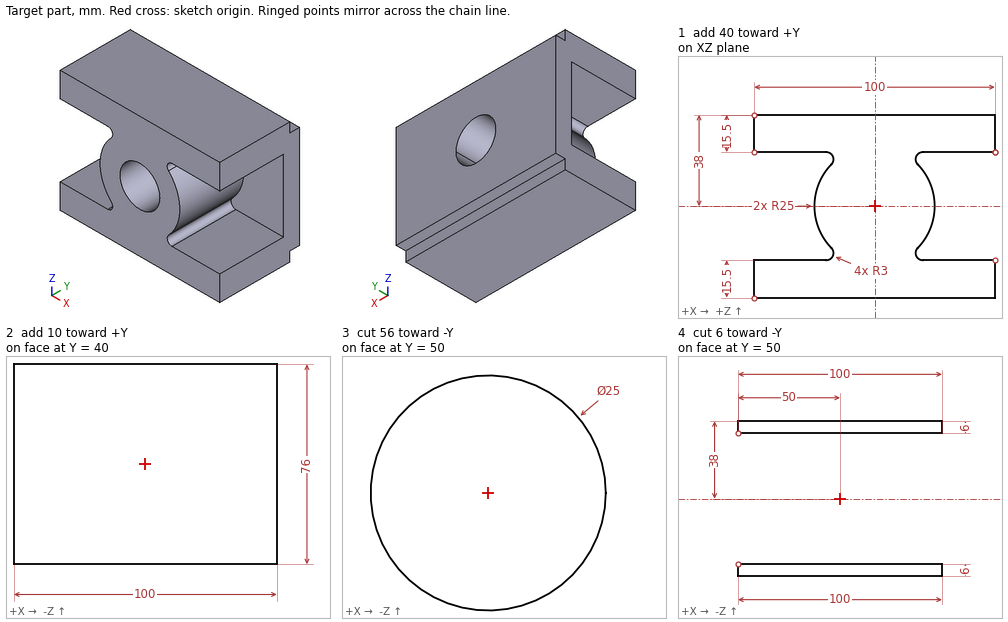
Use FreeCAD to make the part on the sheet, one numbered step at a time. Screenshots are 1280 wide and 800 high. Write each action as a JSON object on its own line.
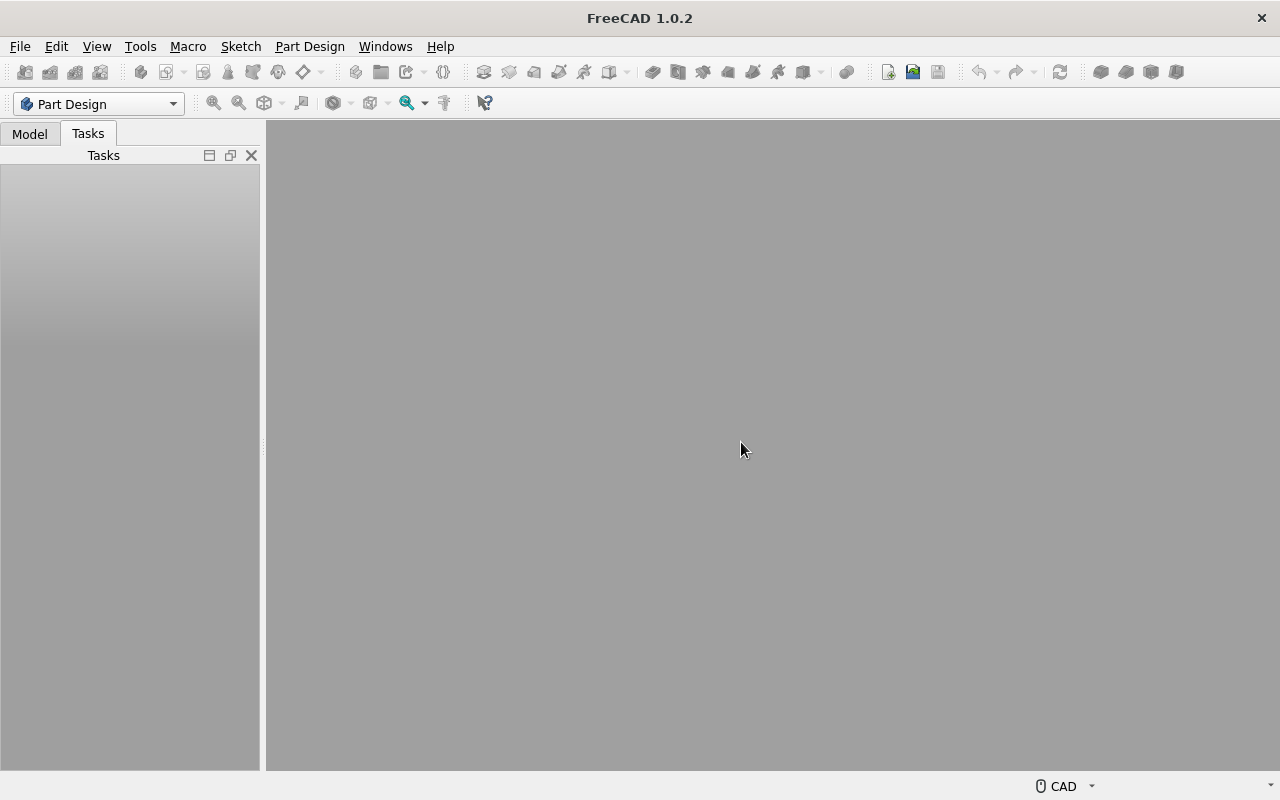
{"action": "left_click", "coordinate": [888, 72]}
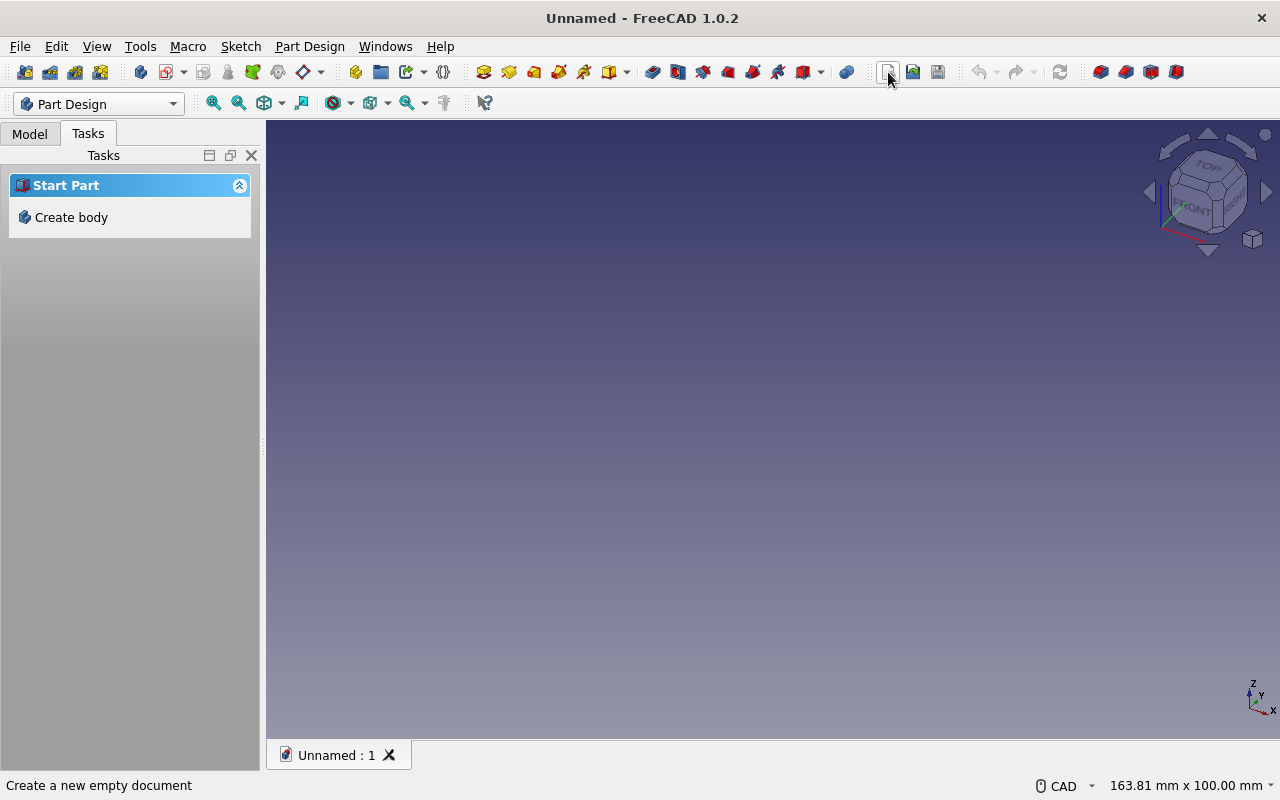
{"action": "left_click", "coordinate": [166, 72]}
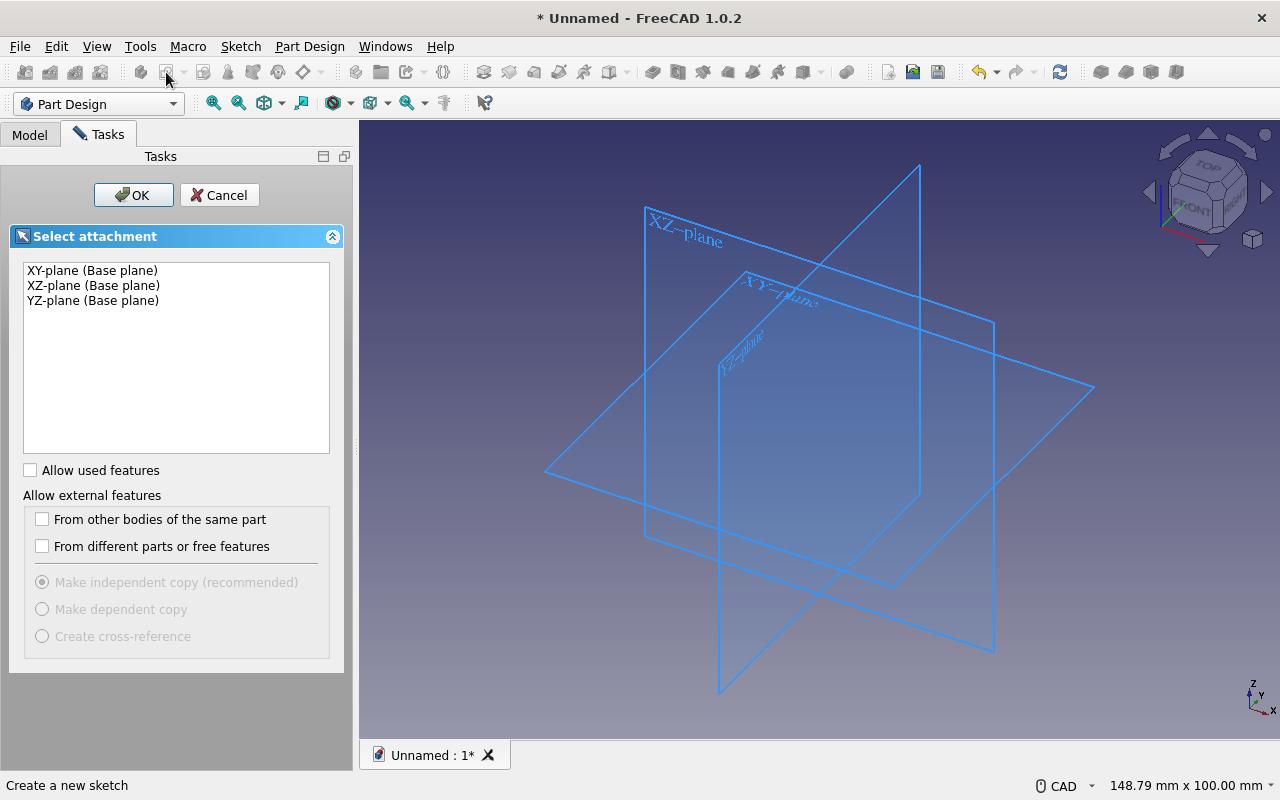
{"action": "left_click", "coordinate": [84, 286]}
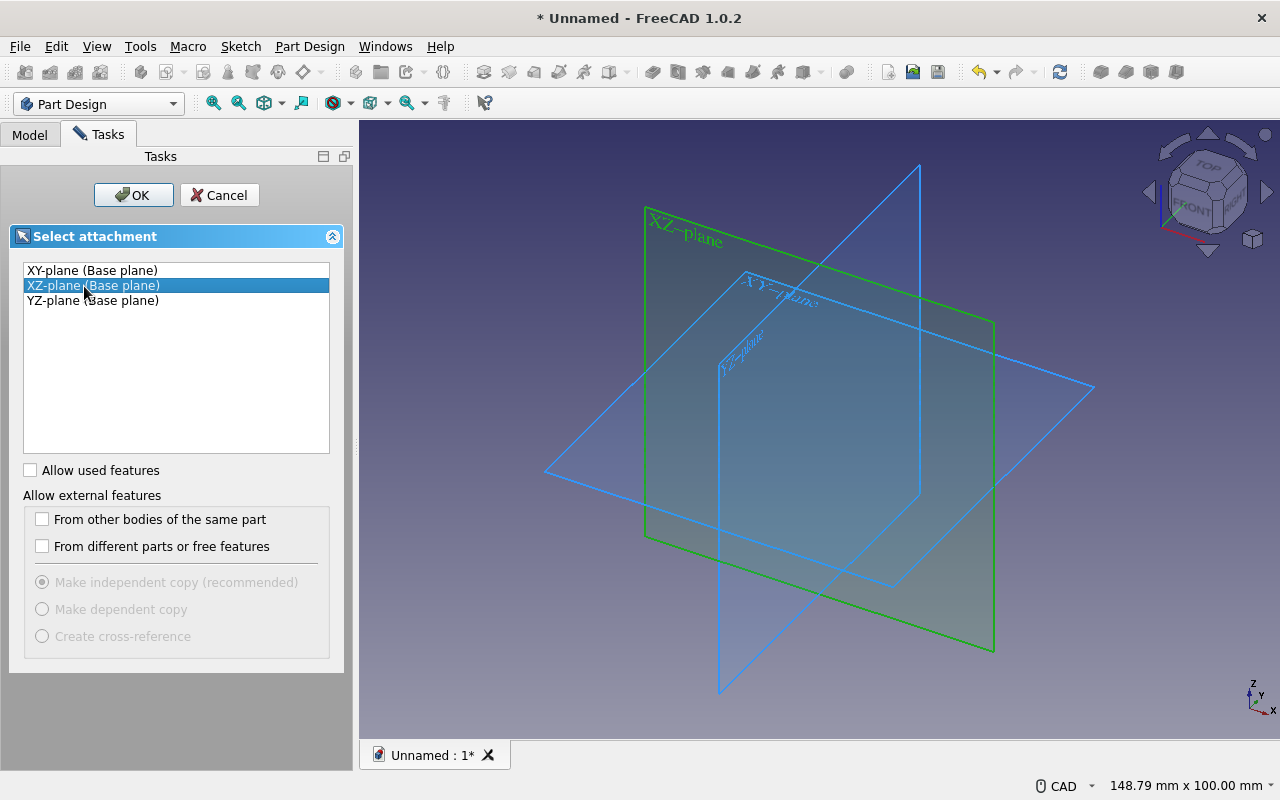
{"action": "left_click", "coordinate": [134, 195]}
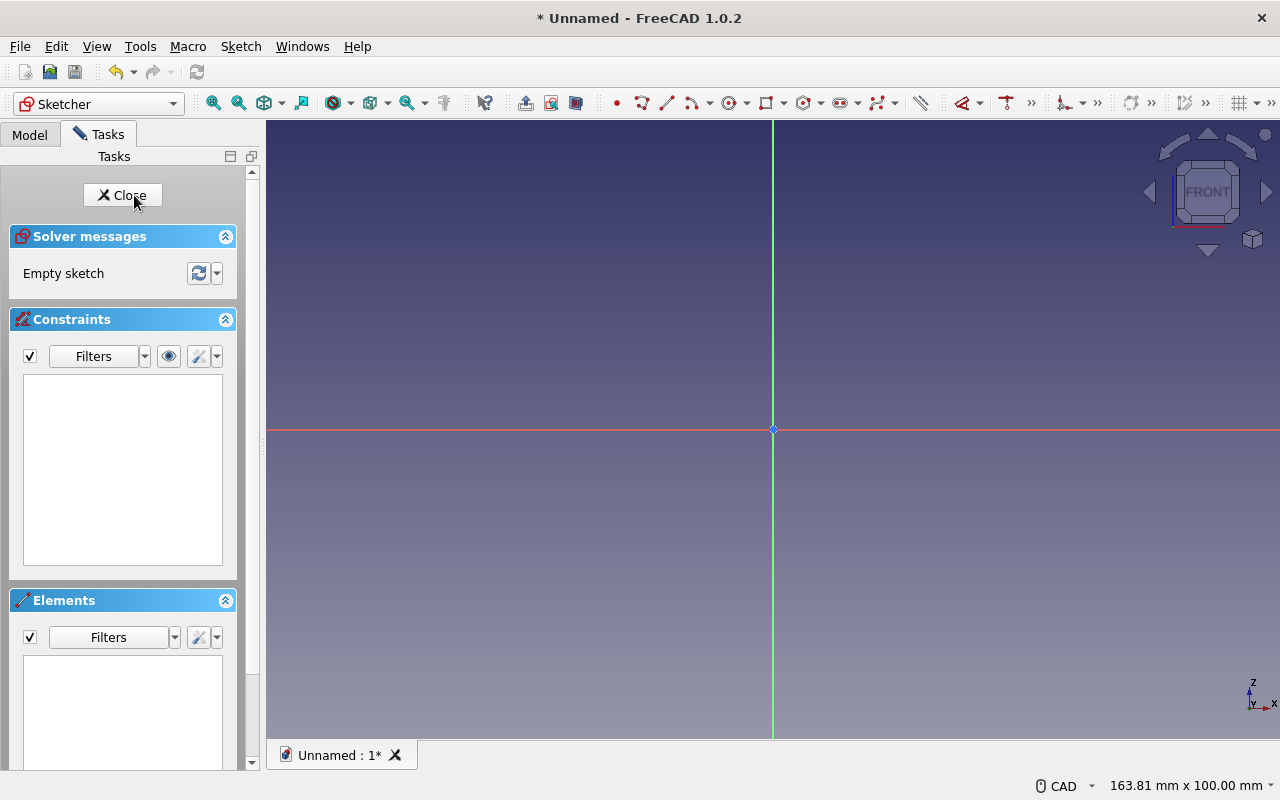
{"action": "left_click", "coordinate": [642, 104]}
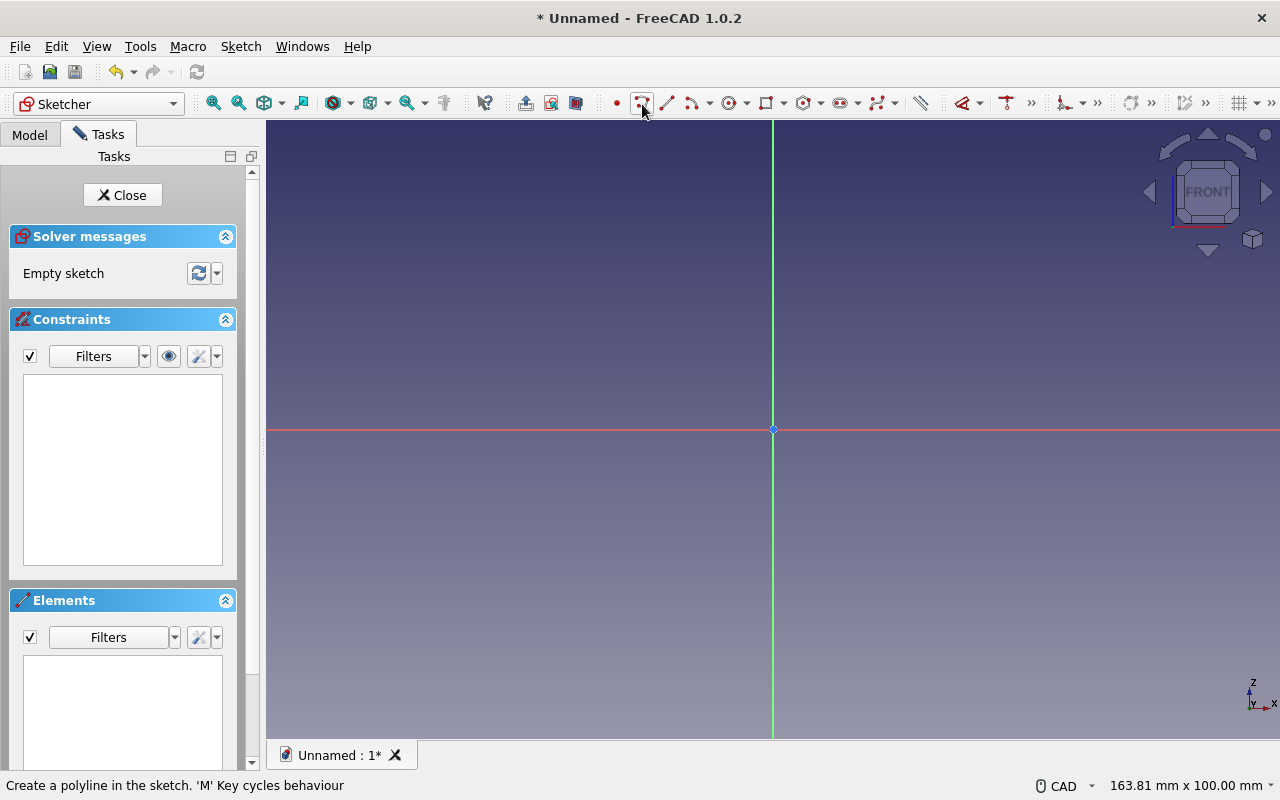
{"action": "left_click", "coordinate": [649, 290]}
{"action": "left_click", "coordinate": [464, 290]}
{"action": "left_click", "coordinate": [464, 194]}
{"action": "left_click", "coordinate": [1082, 194]}
{"action": "left_click", "coordinate": [1082, 290]}
{"action": "left_click", "coordinate": [897, 290]}
{"action": "right_click", "coordinate": [897, 290]}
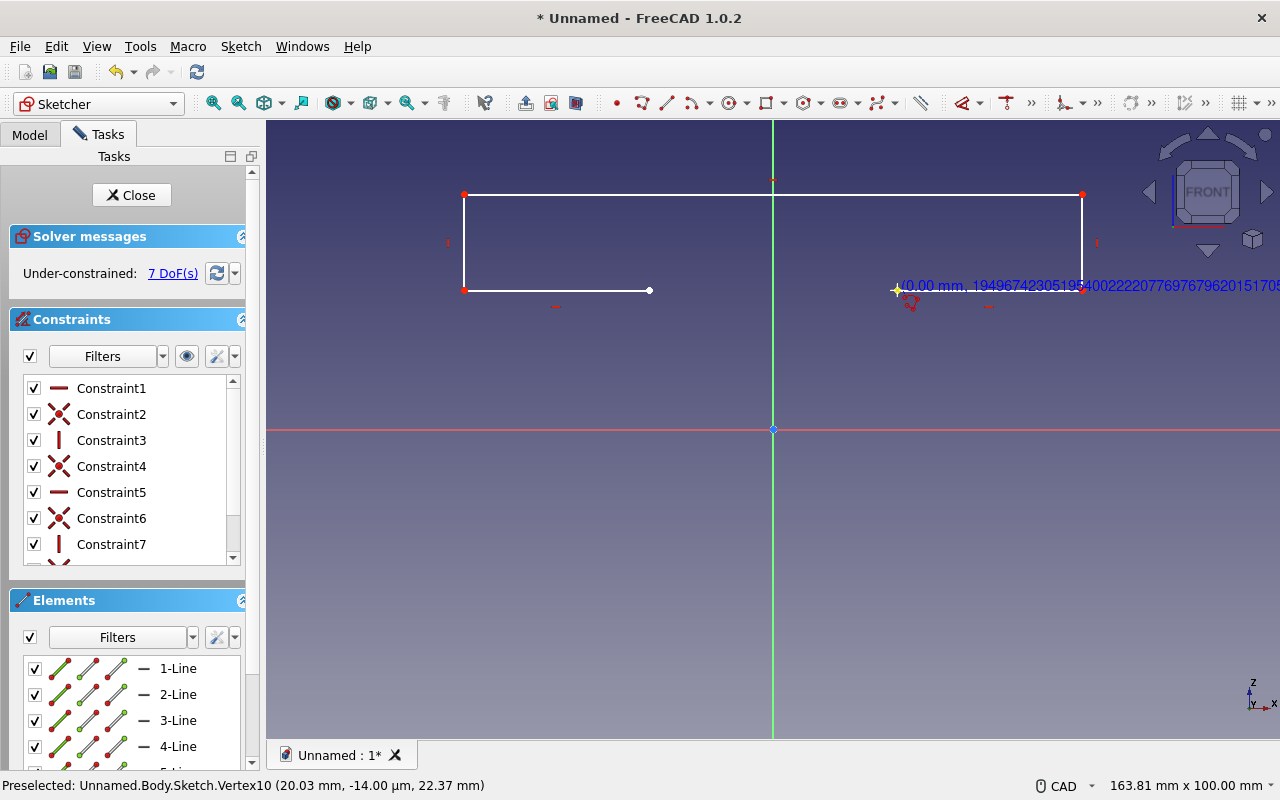
{"action": "left_click", "coordinate": [897, 569]}
{"action": "left_click", "coordinate": [1082, 569]}
{"action": "left_click", "coordinate": [1082, 665]}
{"action": "left_click", "coordinate": [464, 665]}
{"action": "left_click", "coordinate": [464, 569]}
{"action": "left_click", "coordinate": [649, 569]}
{"action": "right_click", "coordinate": [649, 569]}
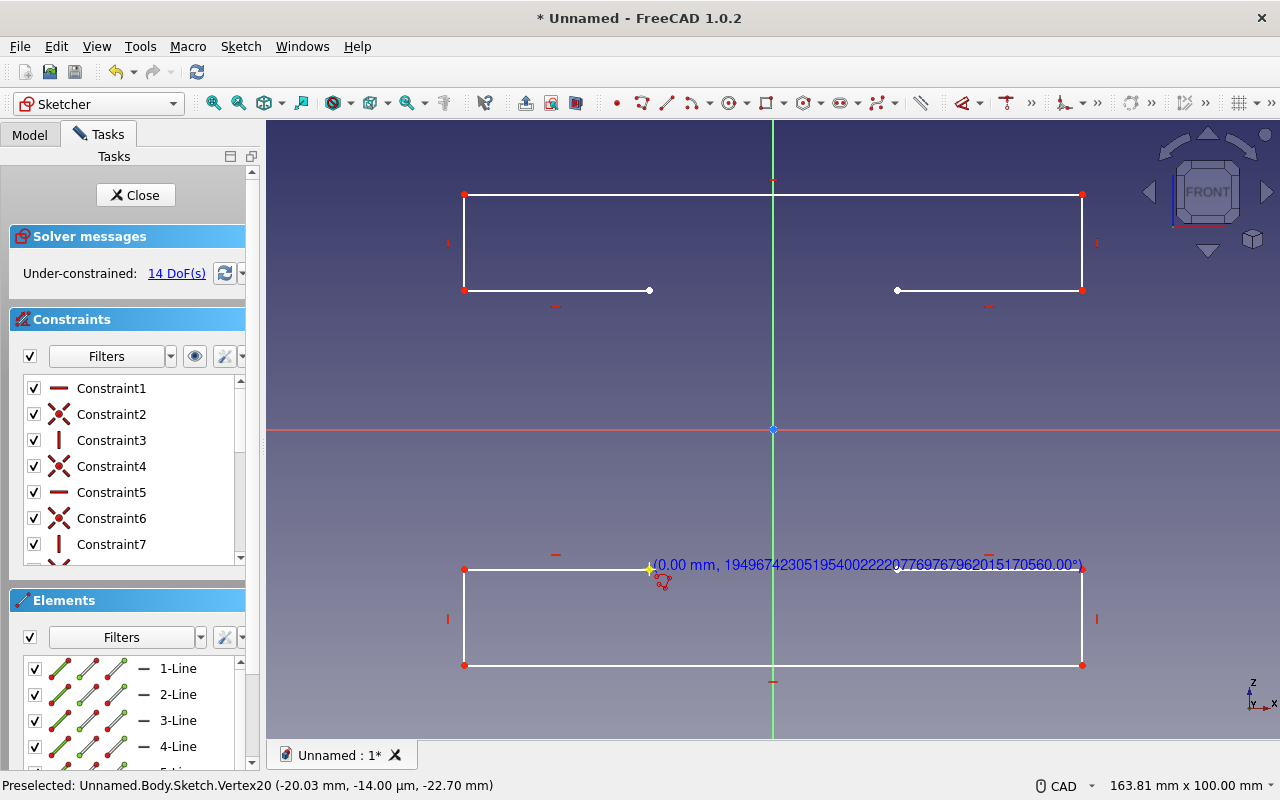
{"action": "left_click", "coordinate": [710, 104]}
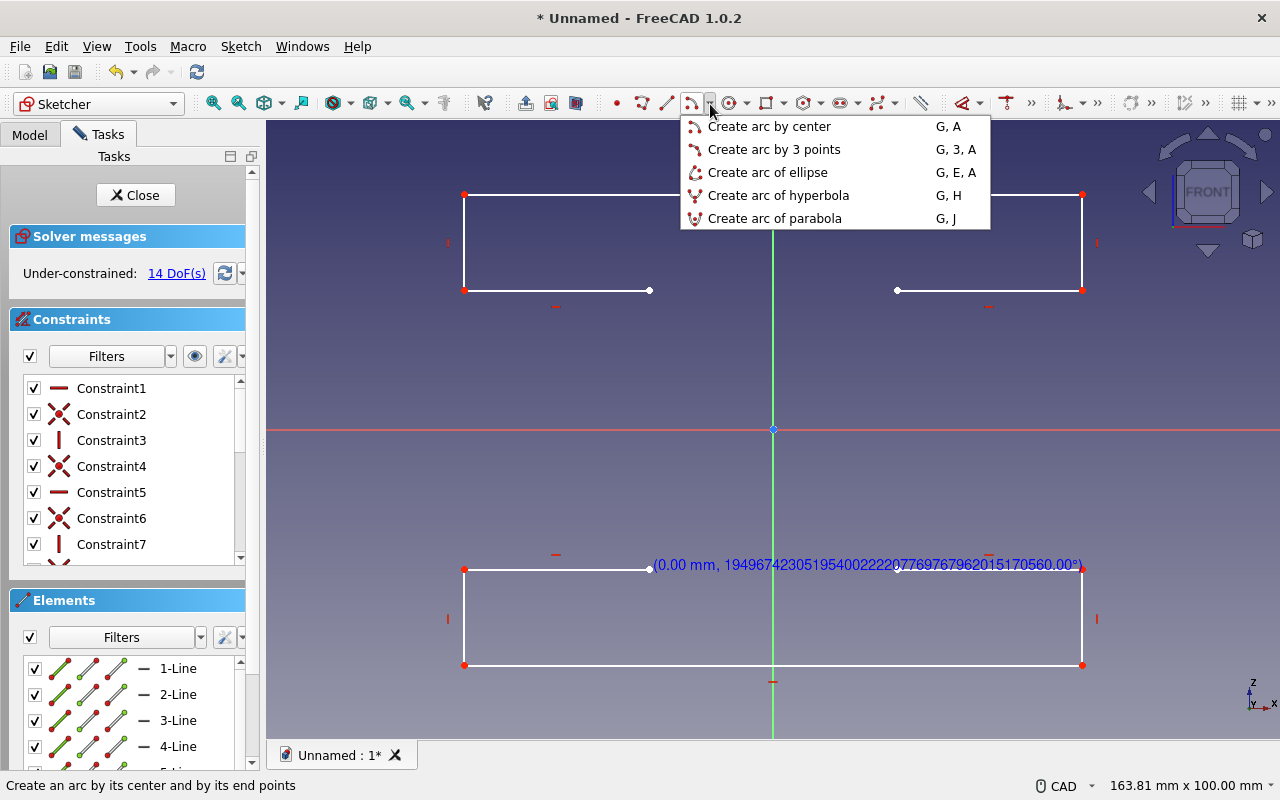
{"action": "left_click", "coordinate": [836, 150]}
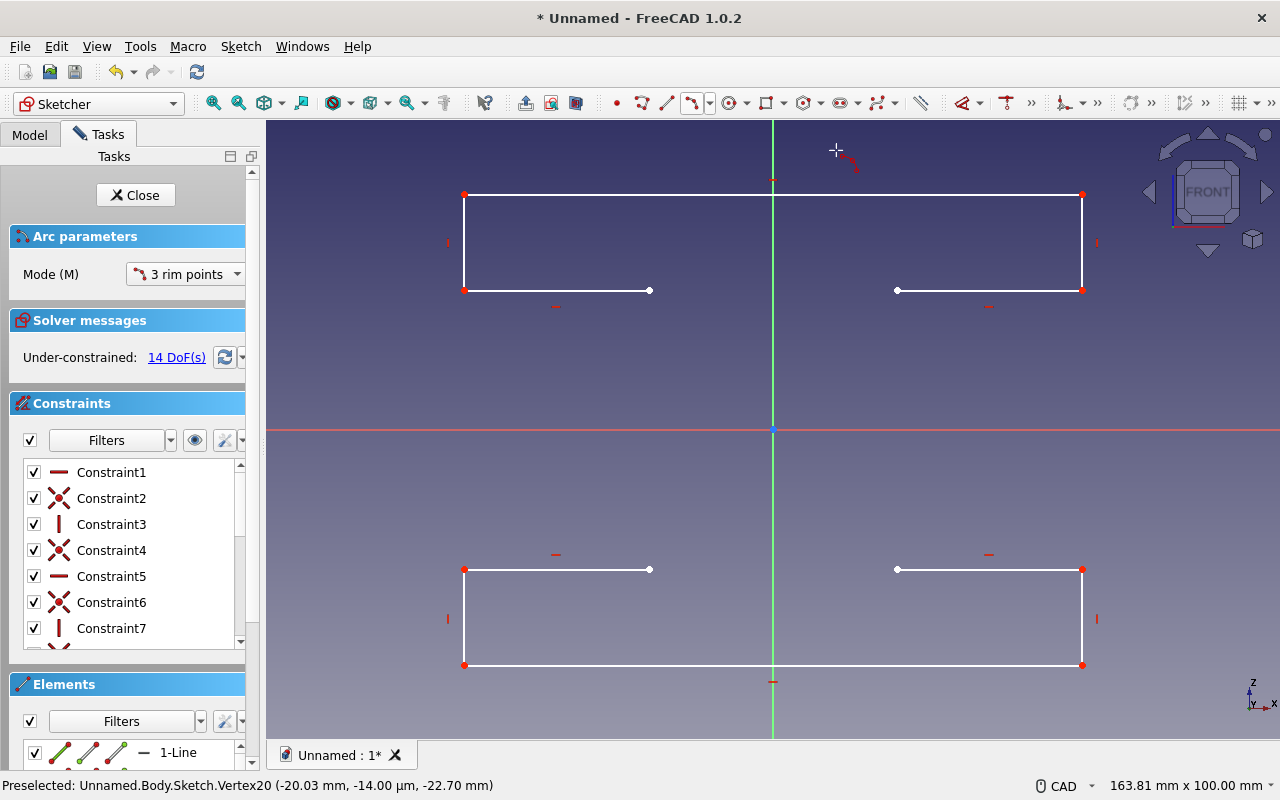
{"action": "left_click", "coordinate": [897, 291]}
{"action": "left_click", "coordinate": [884, 322]}